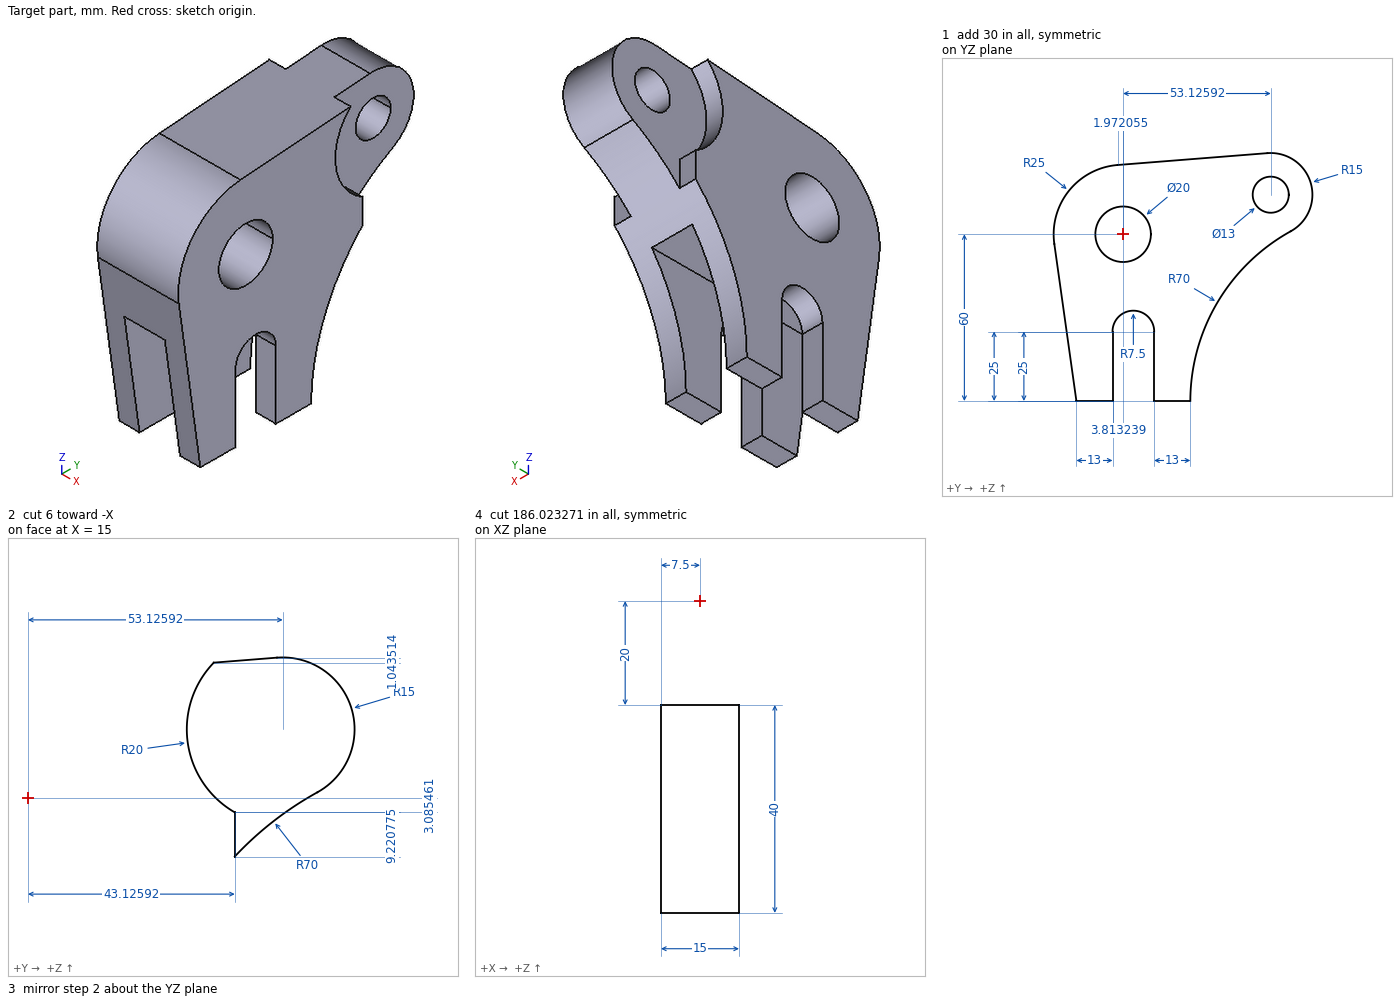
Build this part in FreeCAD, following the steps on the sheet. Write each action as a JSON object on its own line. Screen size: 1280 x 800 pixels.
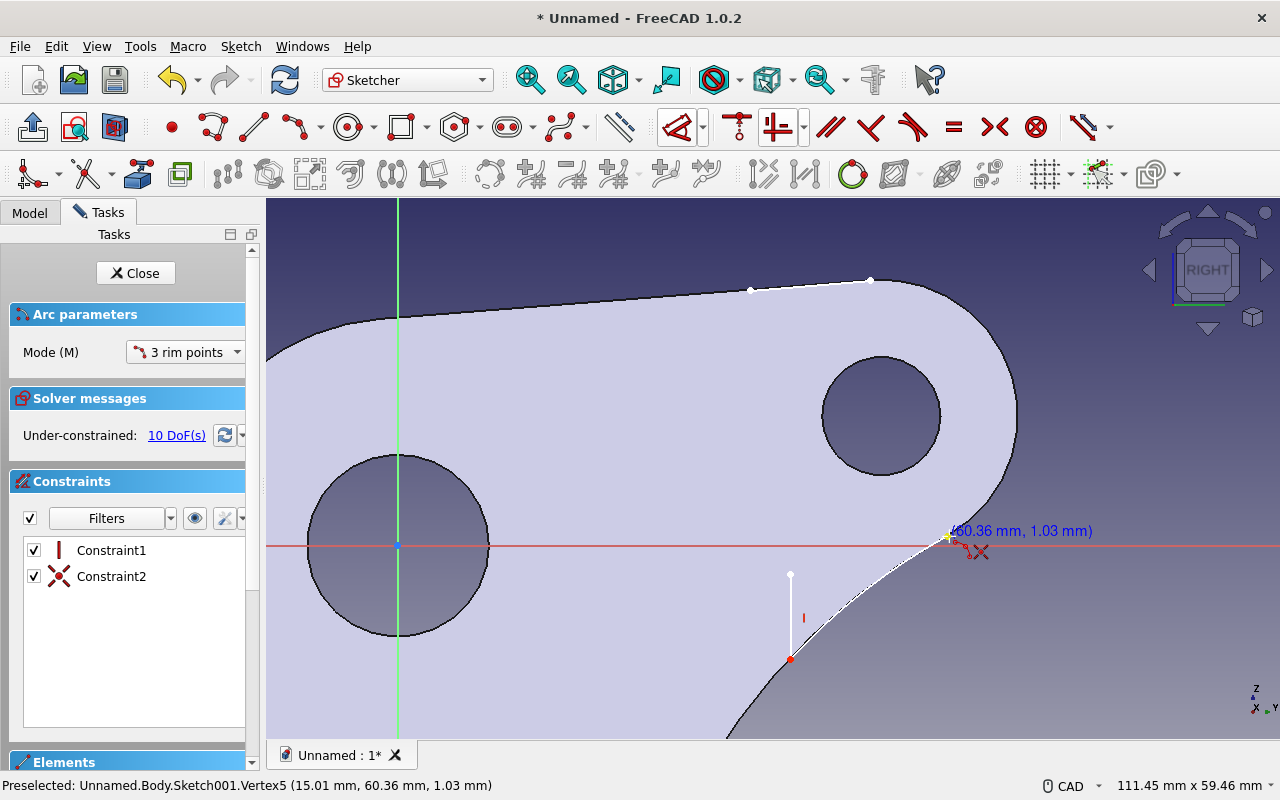
{"action": "left_click", "coordinate": [871, 281]}
{"action": "left_click", "coordinate": [1012, 377]}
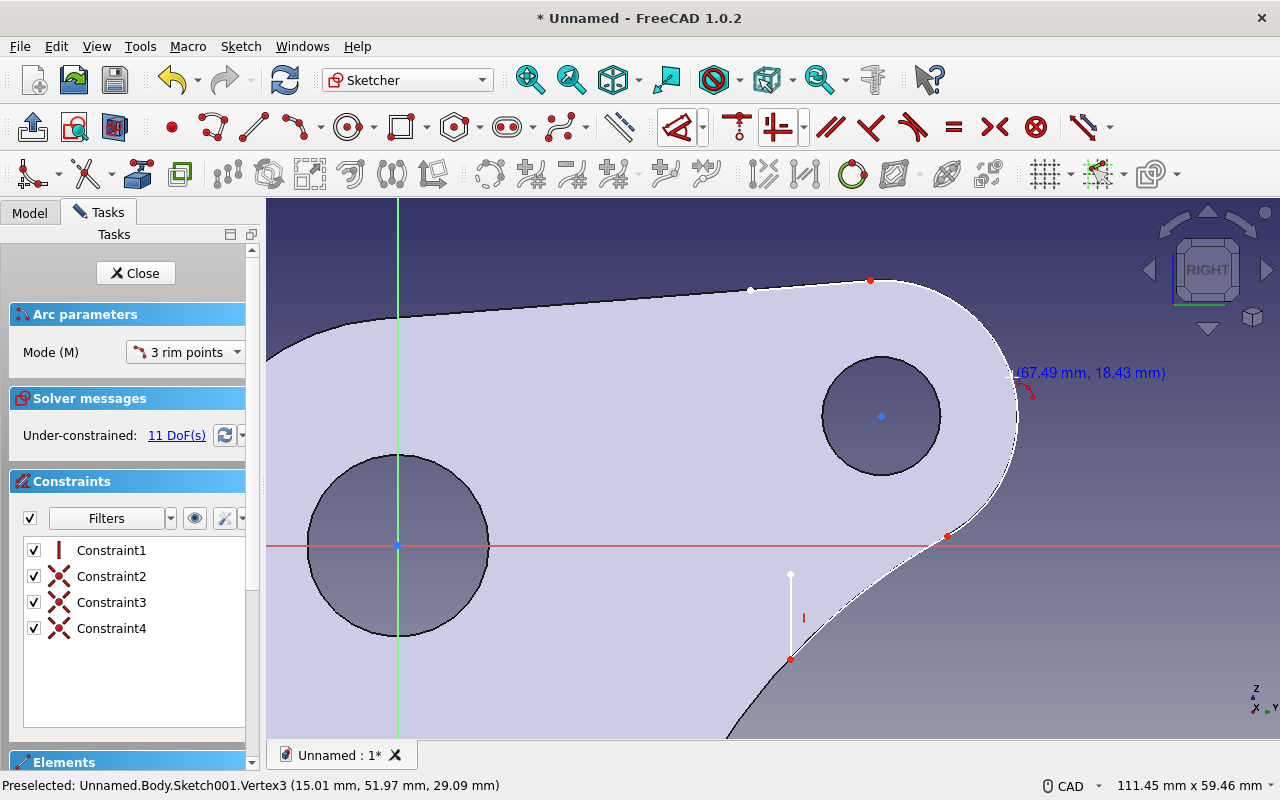
{"action": "left_click", "coordinate": [751, 291]}
{"action": "left_click", "coordinate": [791, 575]}
{"action": "left_click", "coordinate": [701, 441]}
{"action": "key", "text": "Escape"}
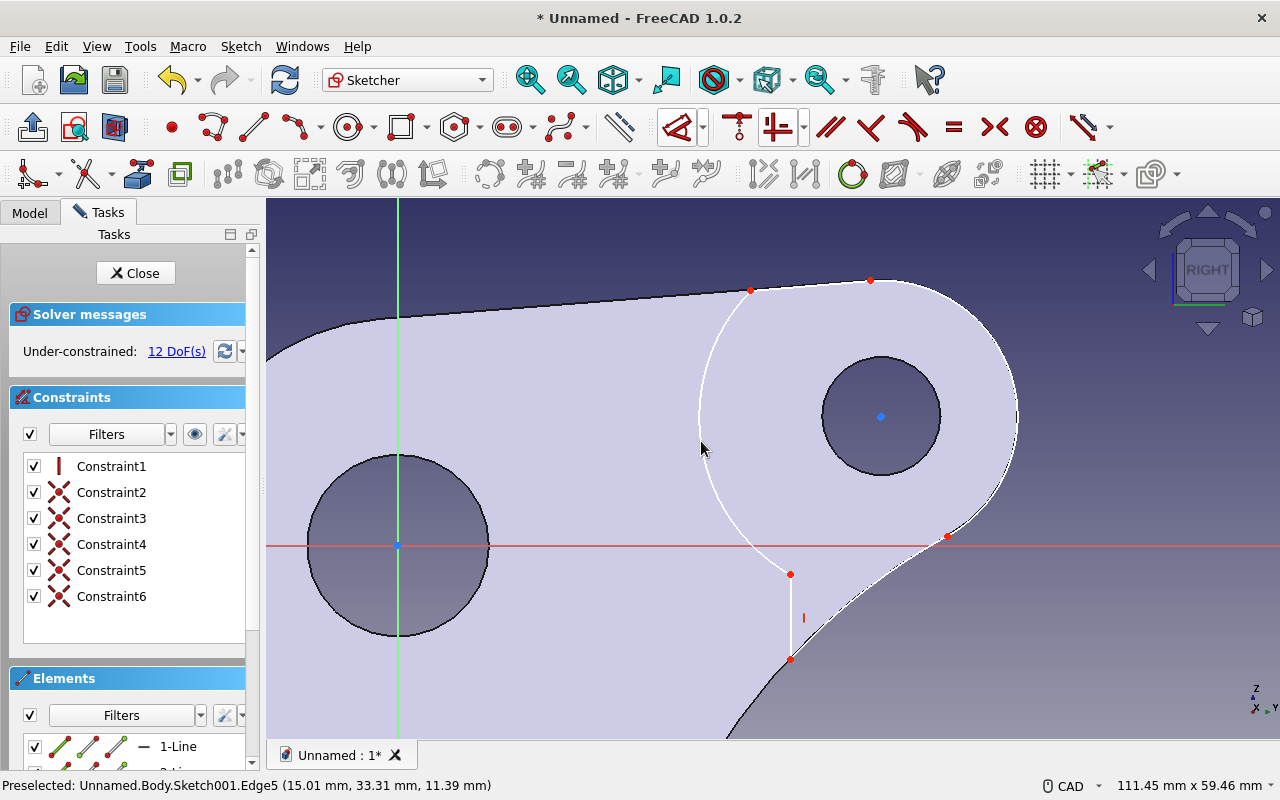
{"action": "left_click", "coordinate": [835, 284]}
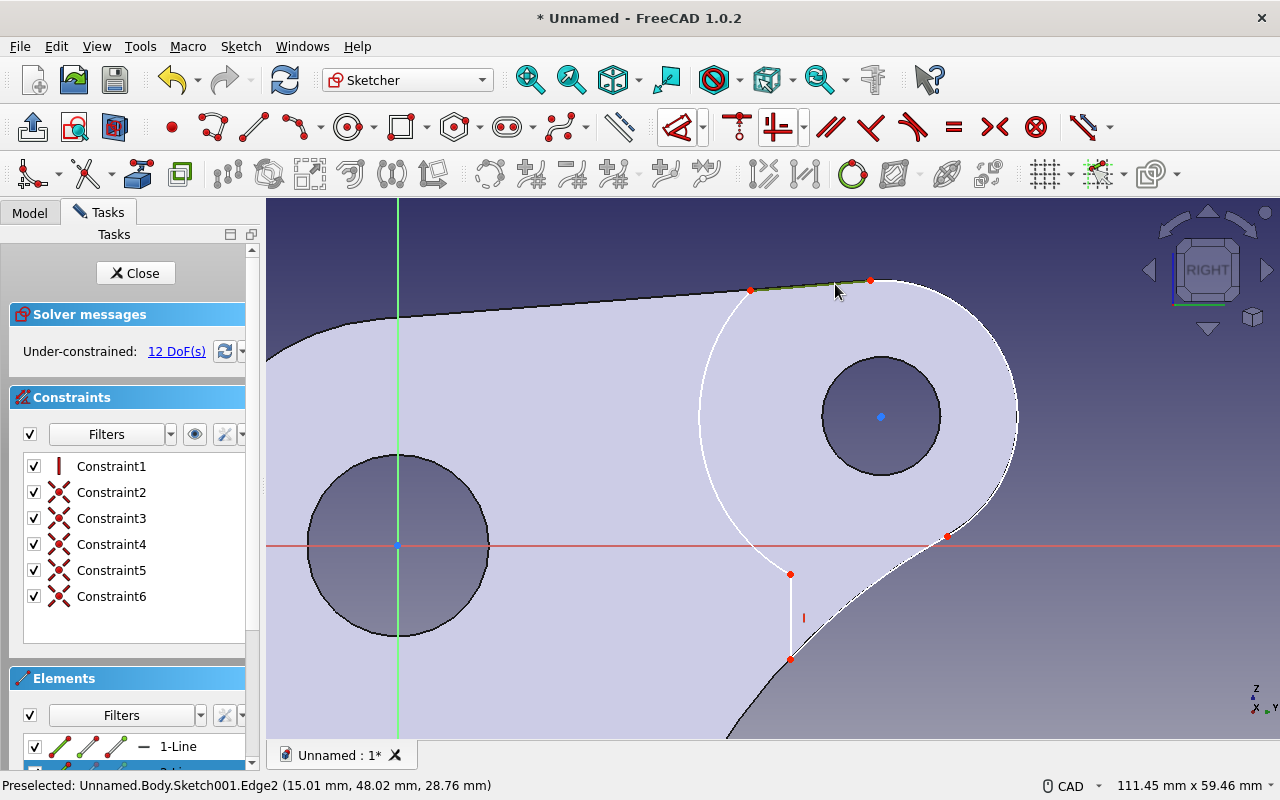
{"action": "left_click", "coordinate": [1013, 451]}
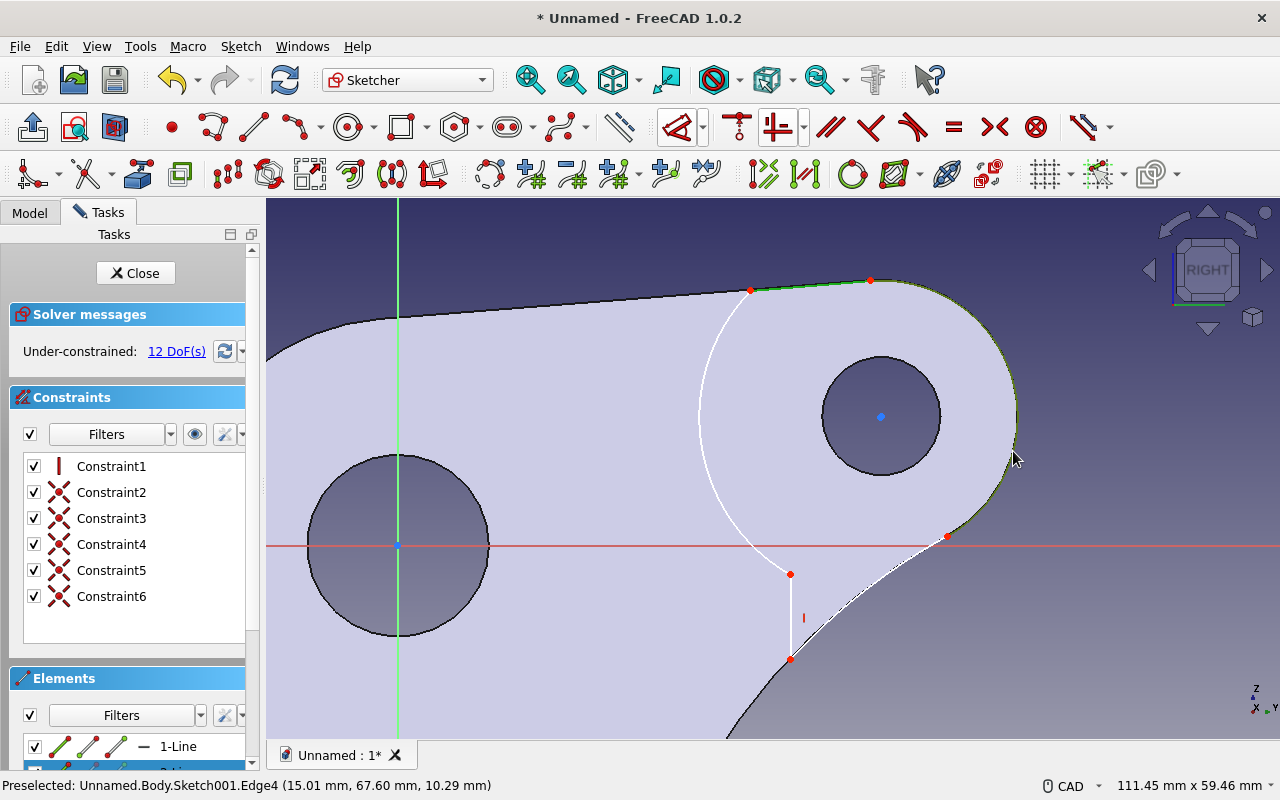
{"action": "left_click", "coordinate": [913, 128]}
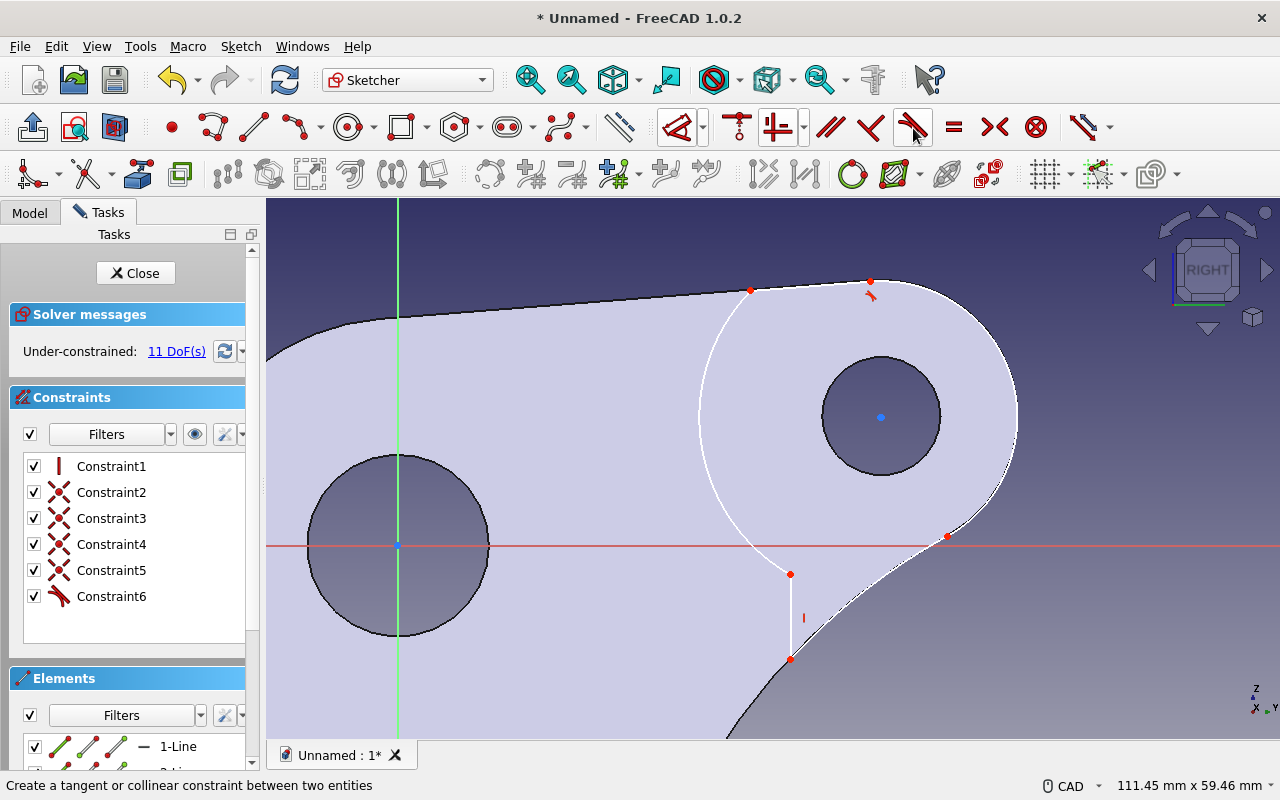
{"action": "left_click", "coordinate": [896, 568]}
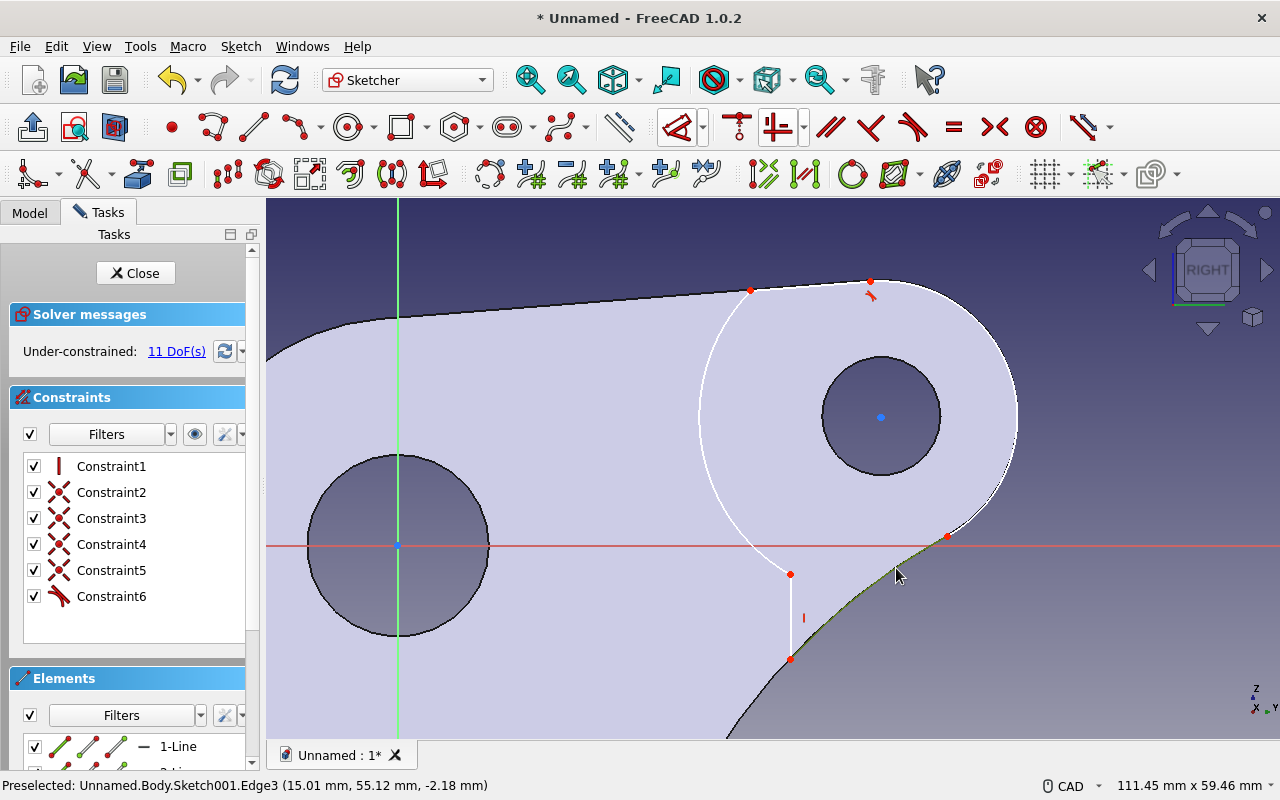
{"action": "left_click", "coordinate": [1013, 451]}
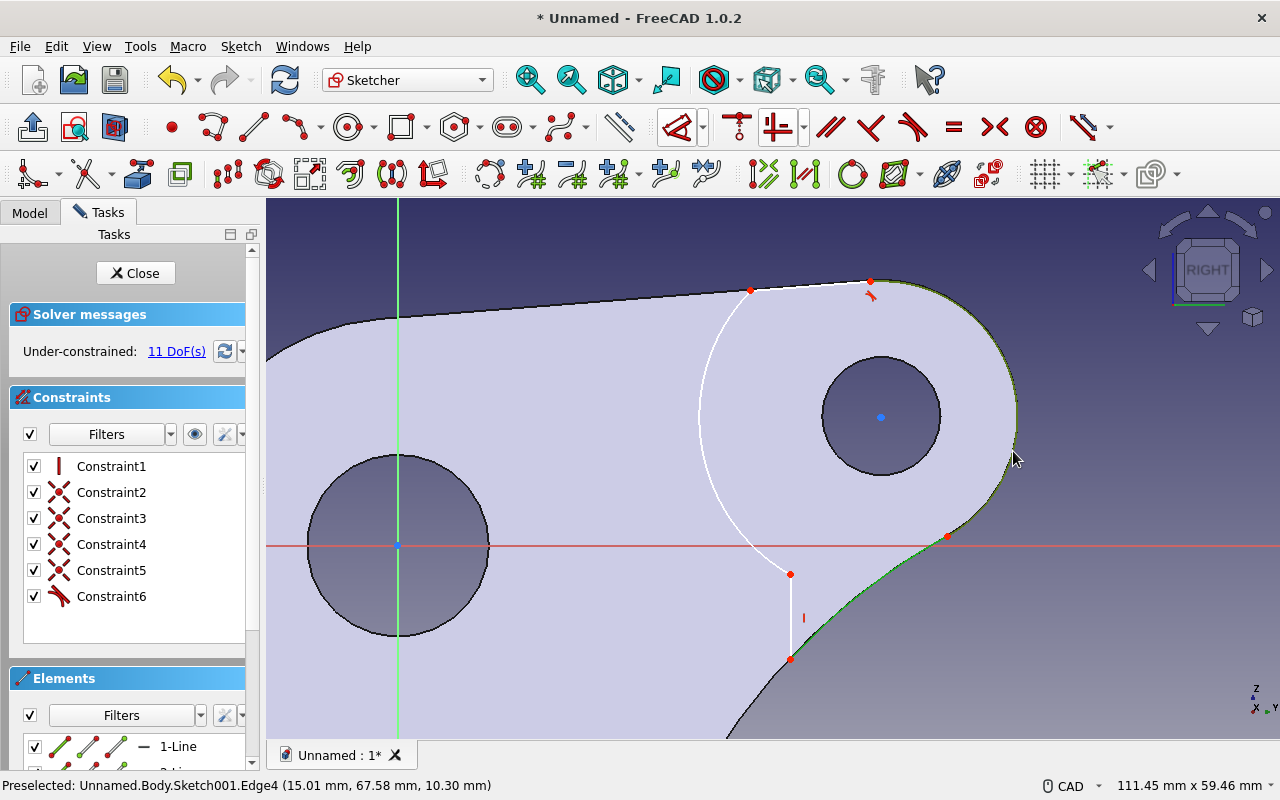
{"action": "left_click", "coordinate": [913, 128]}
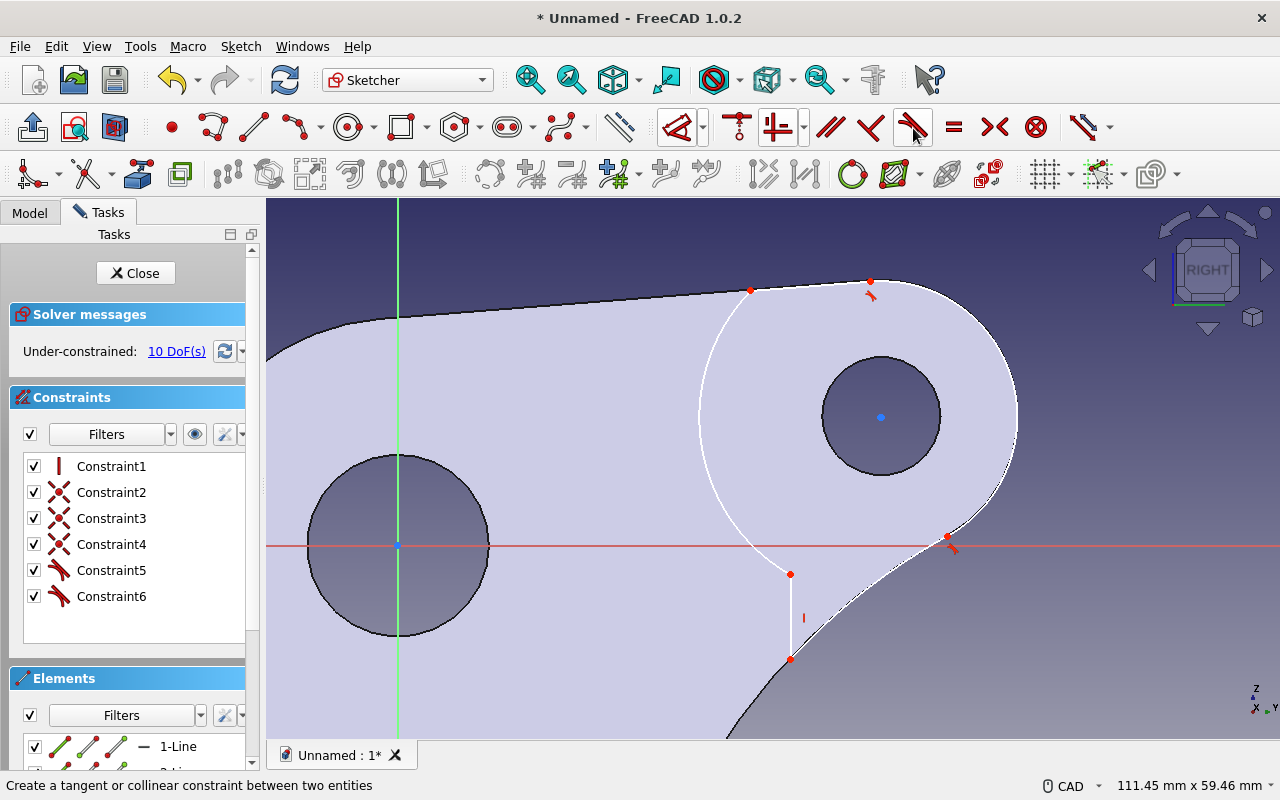
{"action": "left_click", "coordinate": [1013, 451]}